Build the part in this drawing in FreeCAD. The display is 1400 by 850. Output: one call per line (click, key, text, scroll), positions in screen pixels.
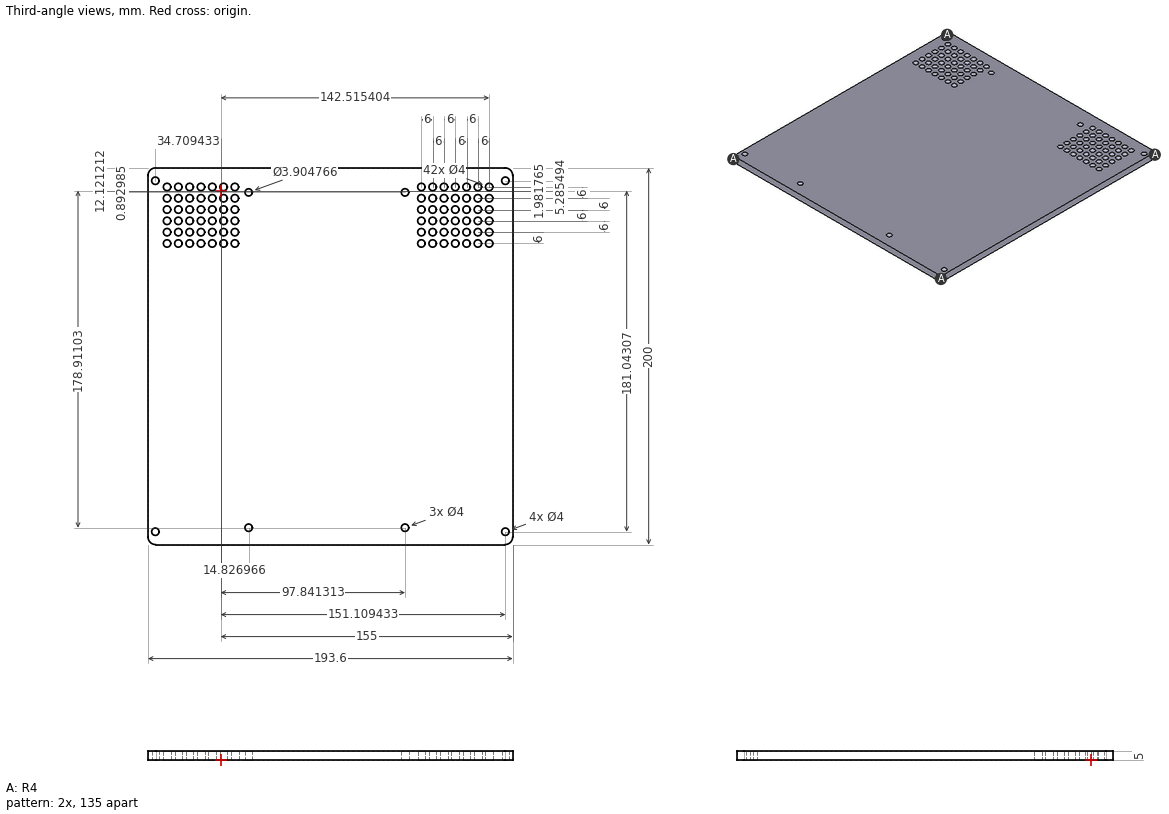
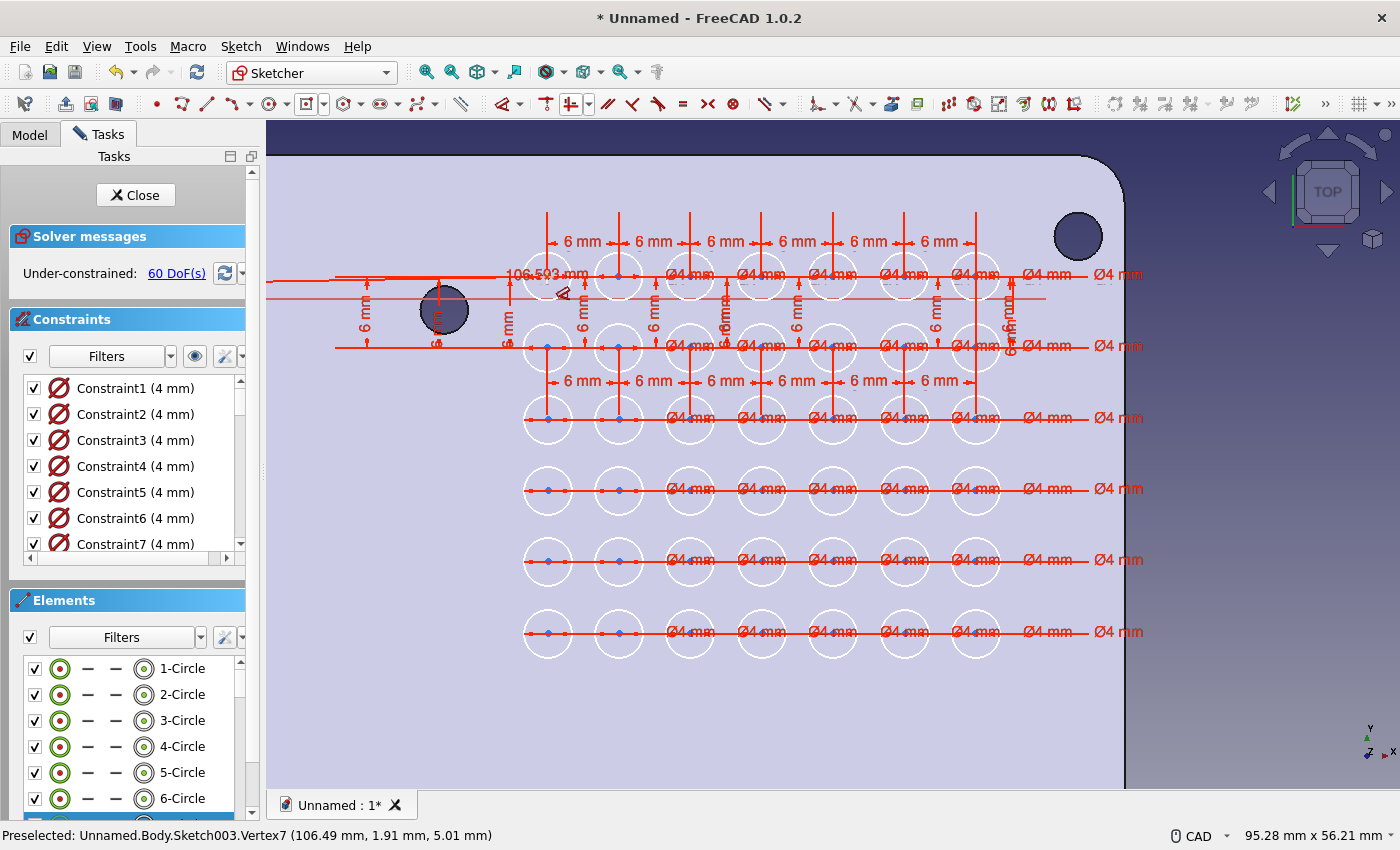
click(547, 348)
click(367, 337)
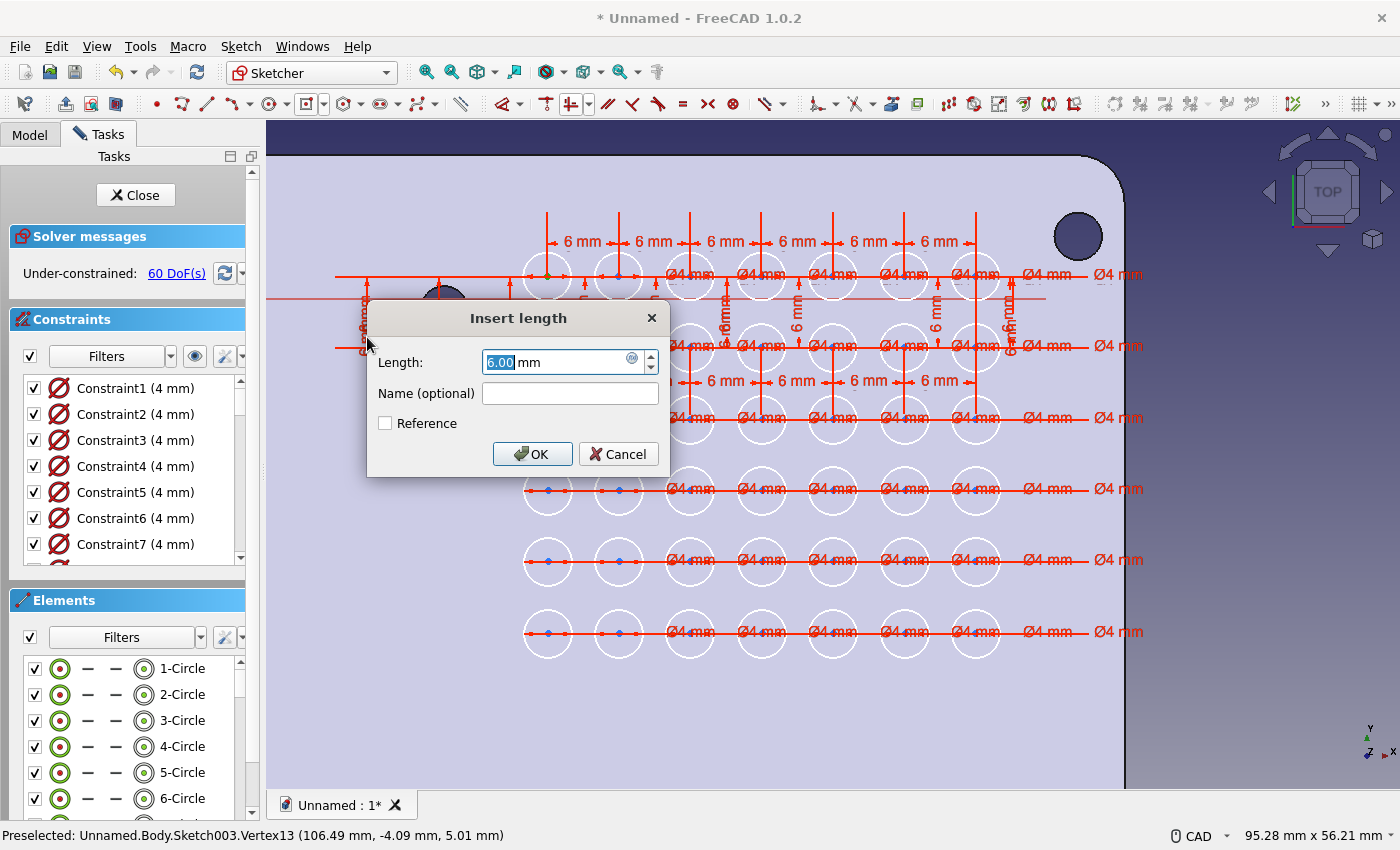
text(6)
key(Return)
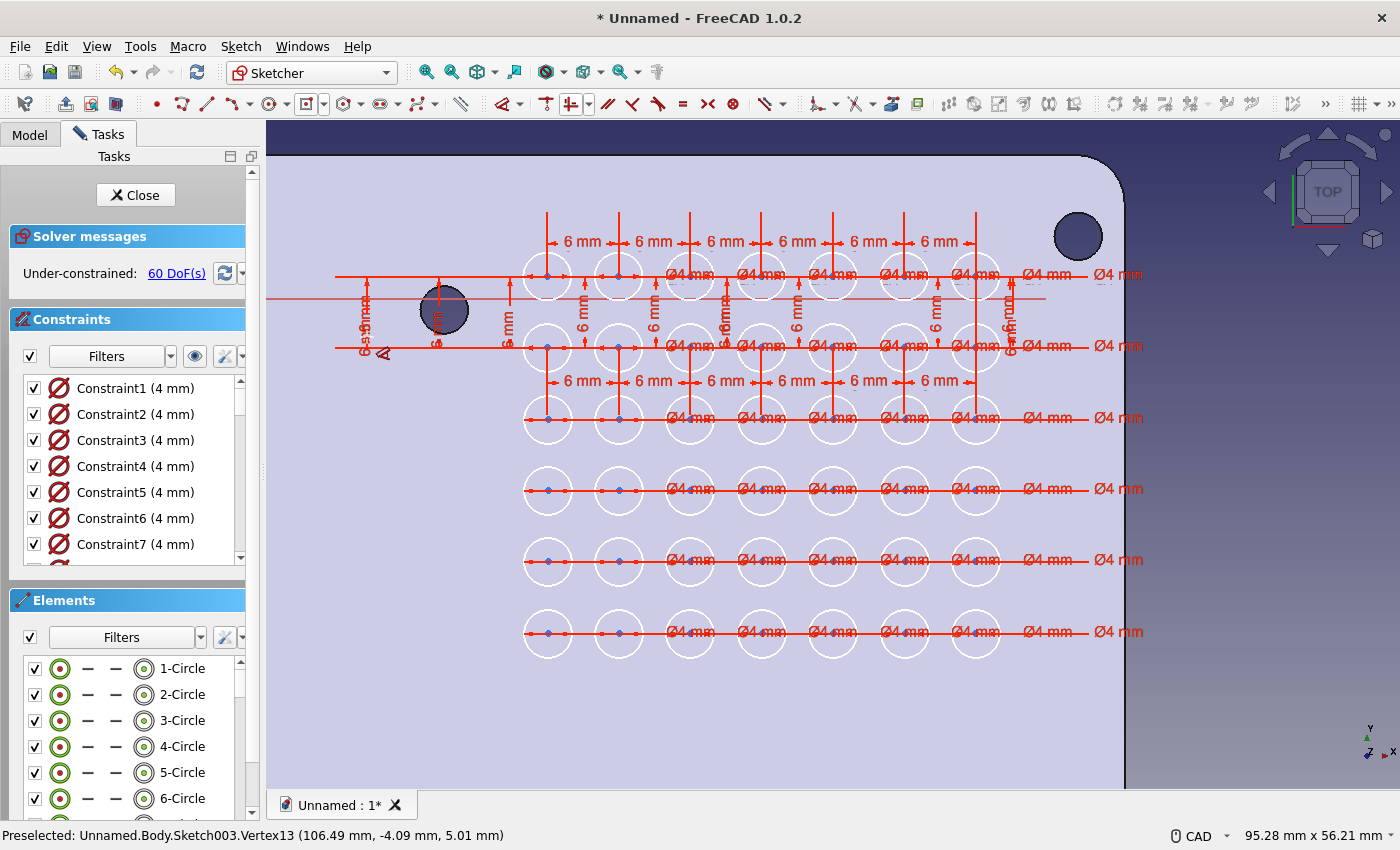
click(833, 348)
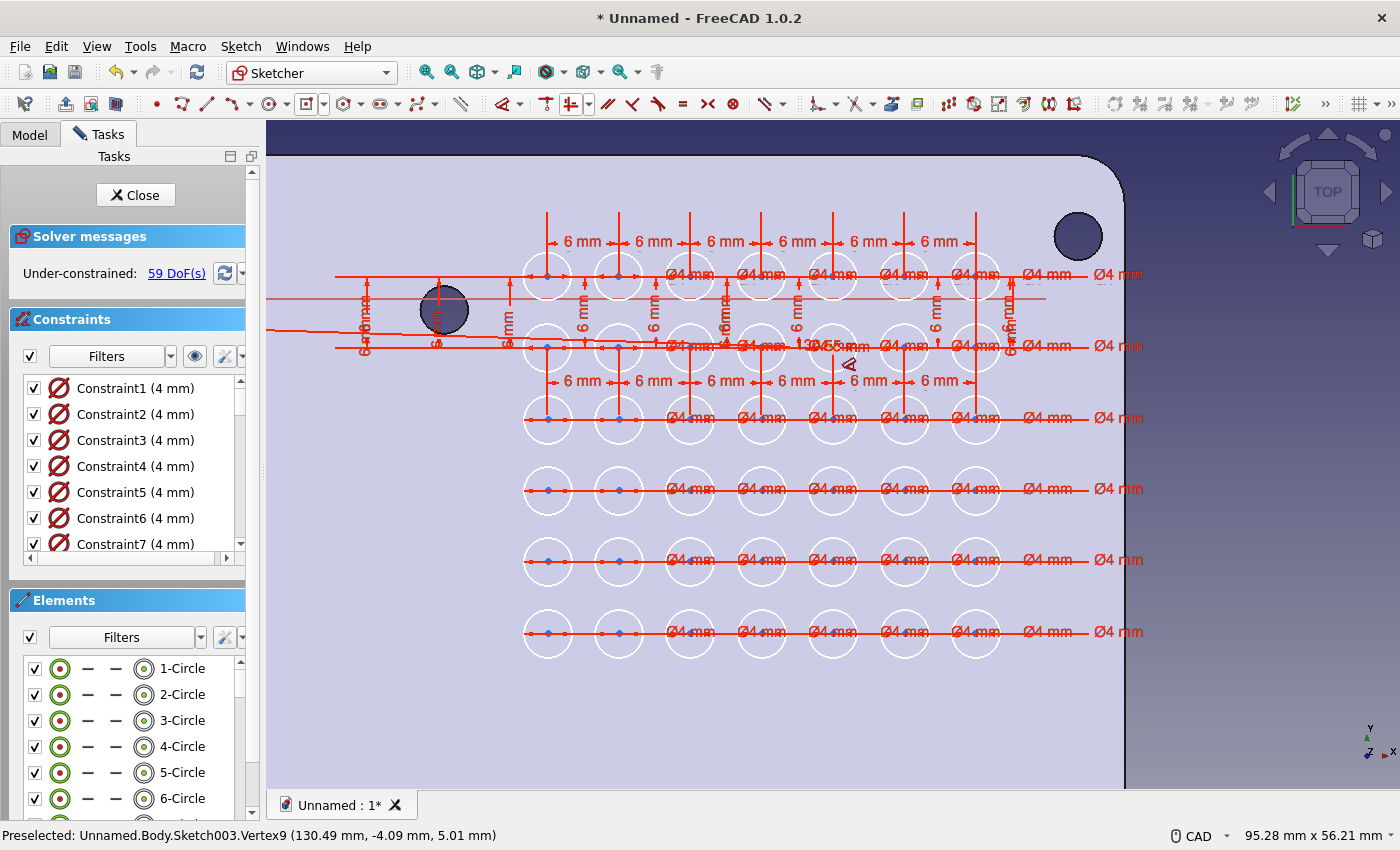
click(905, 420)
click(869, 454)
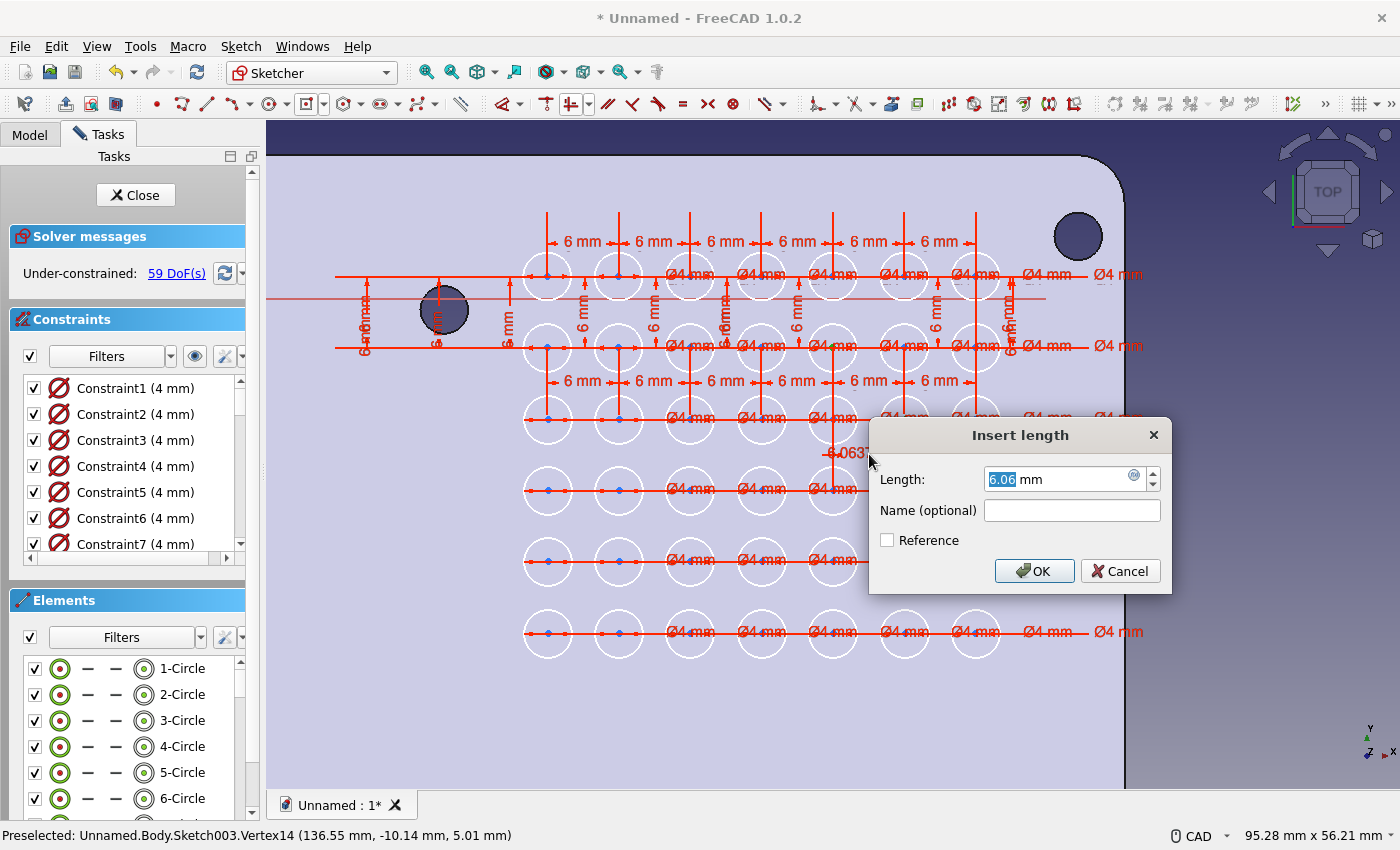
text(6)
key(Return)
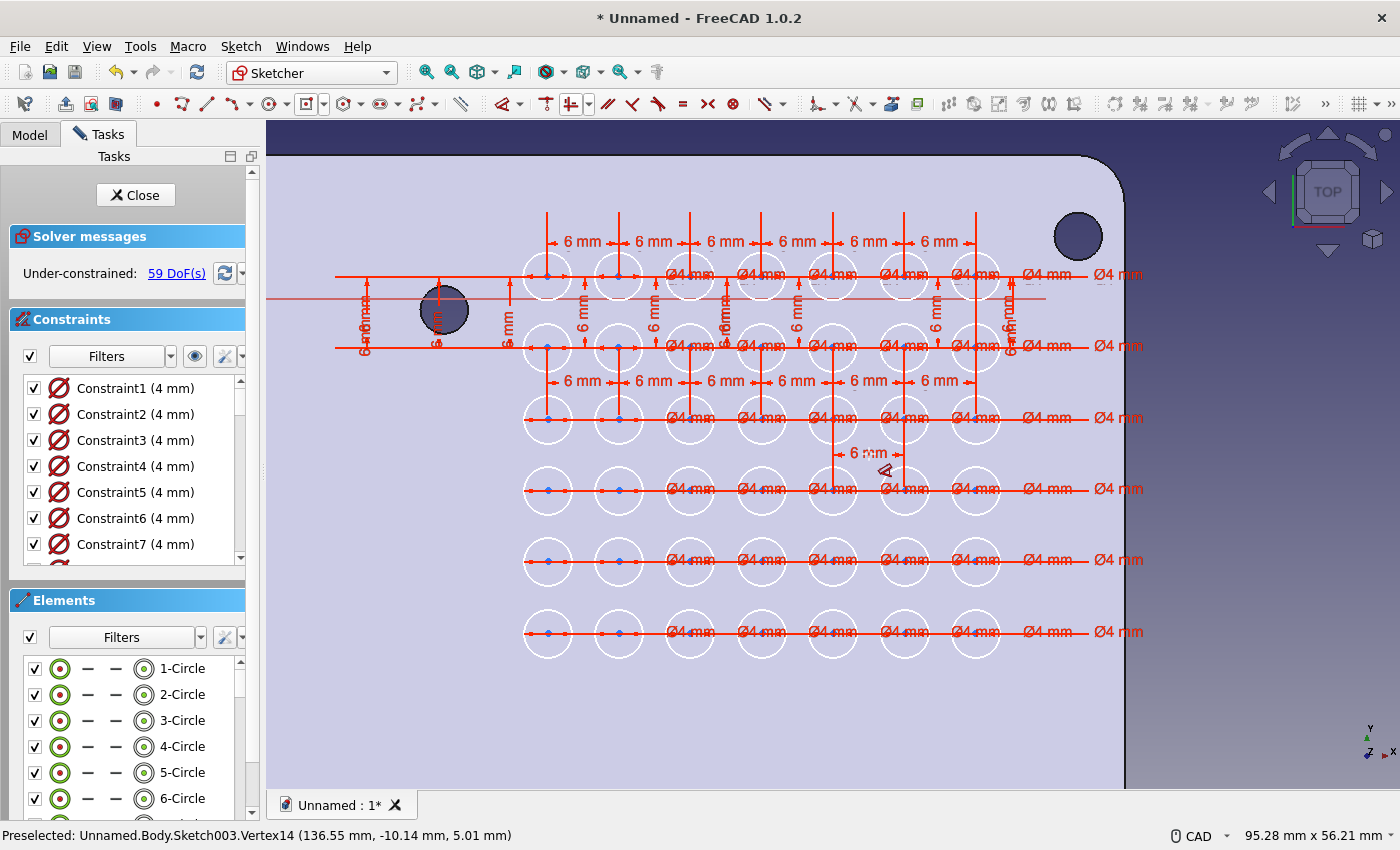
click(904, 348)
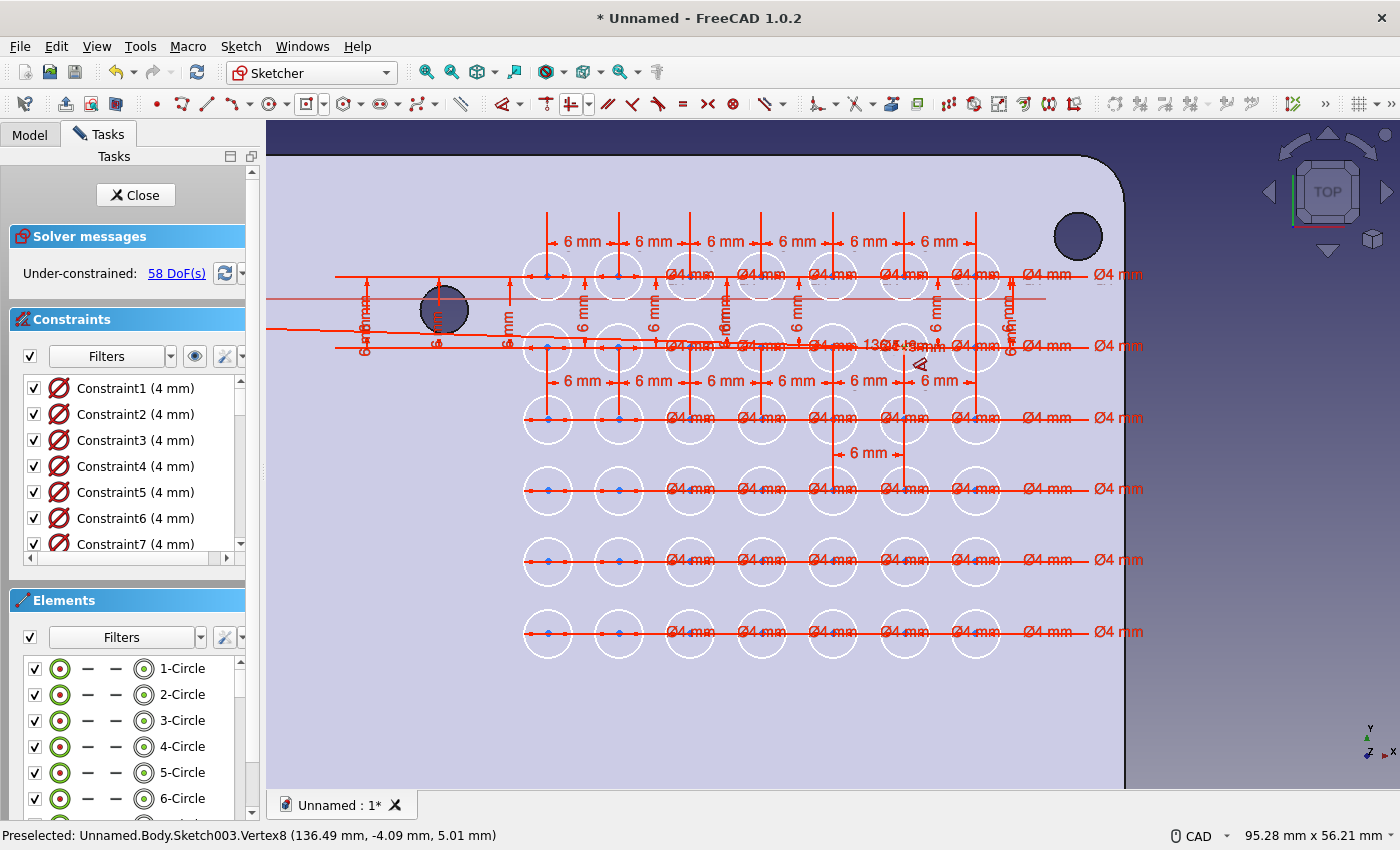
click(904, 420)
click(1034, 384)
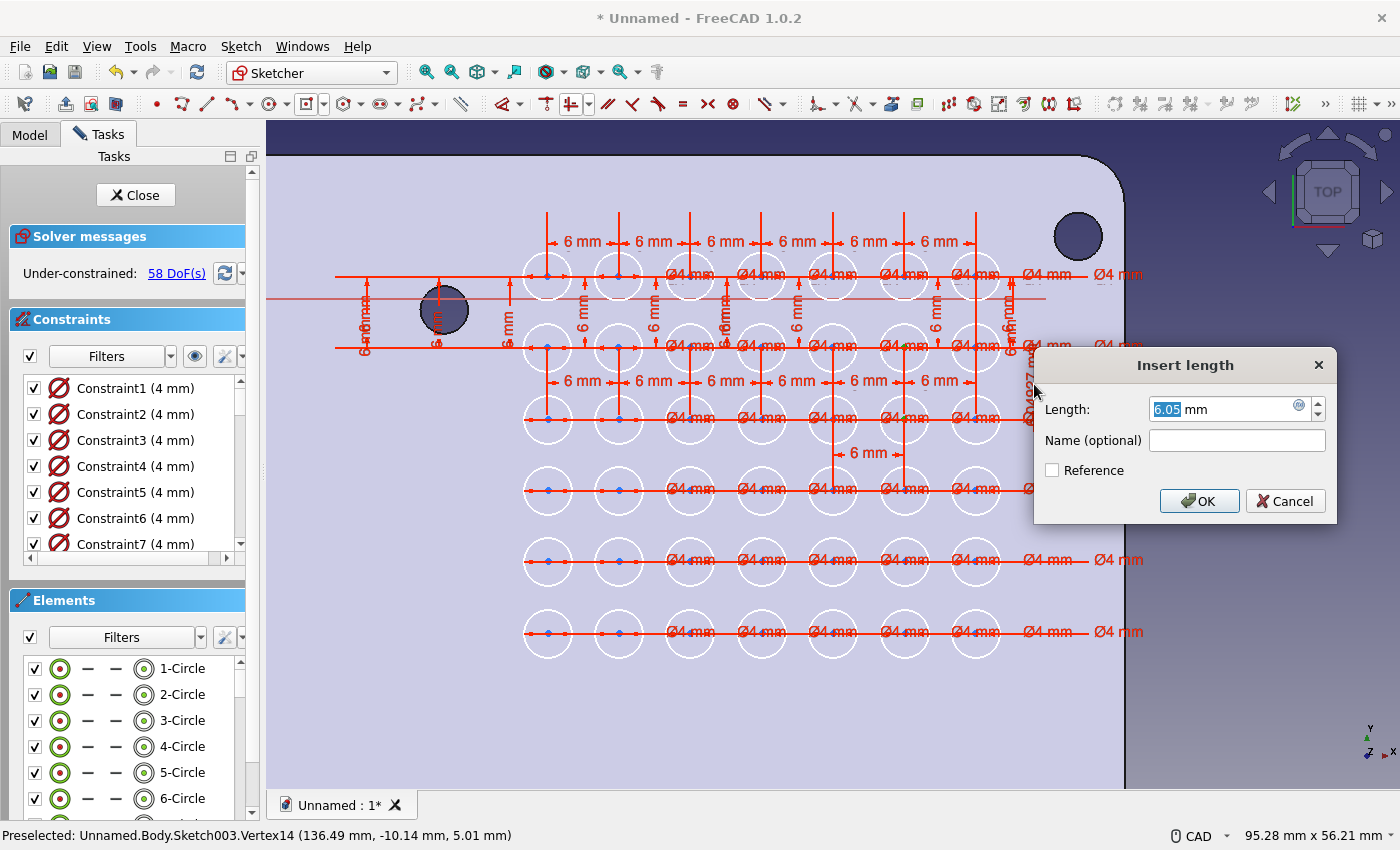
text(6)
key(Return)